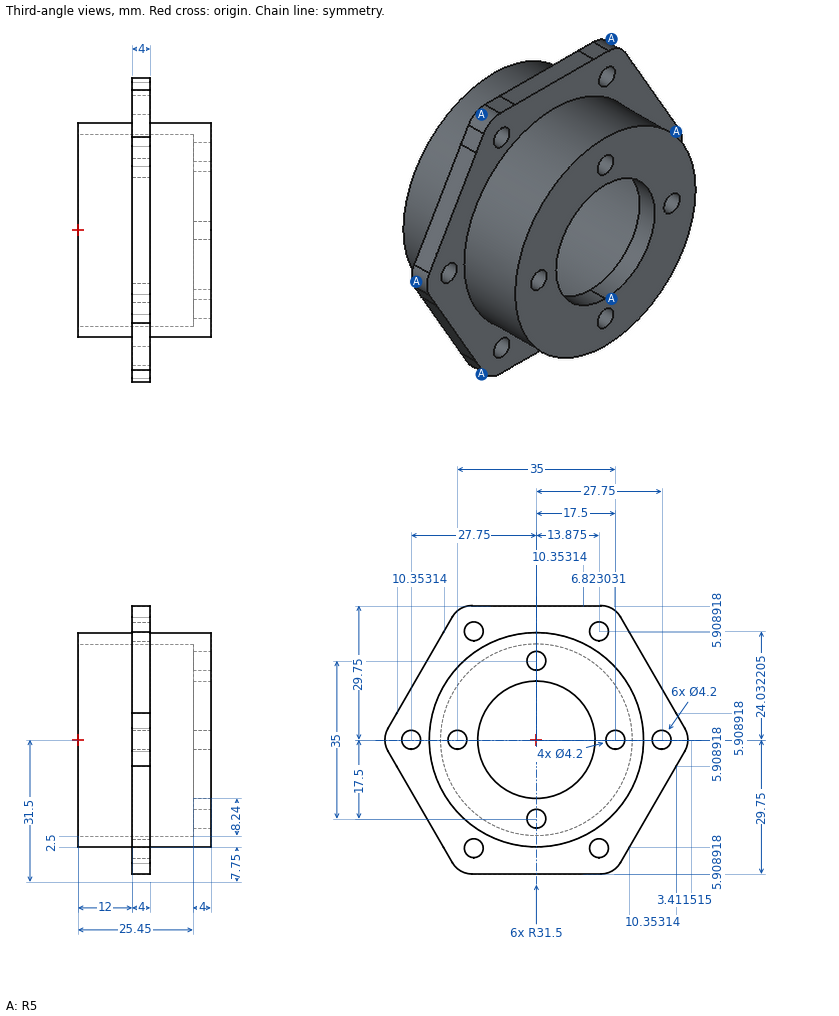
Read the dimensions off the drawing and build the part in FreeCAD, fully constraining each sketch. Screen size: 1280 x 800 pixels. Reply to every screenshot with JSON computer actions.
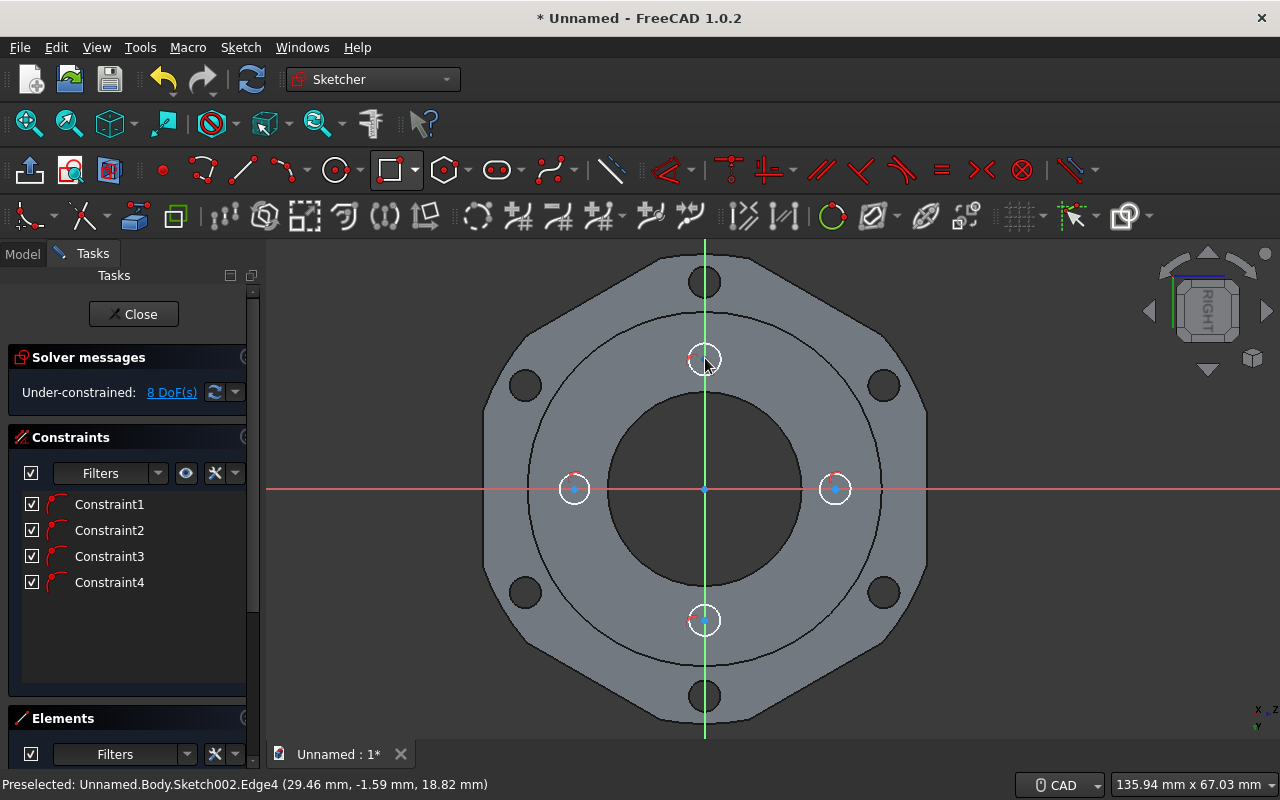
{"action": "scroll", "coordinate": [716, 609], "scroll_direction": "up", "scroll_amount": 2}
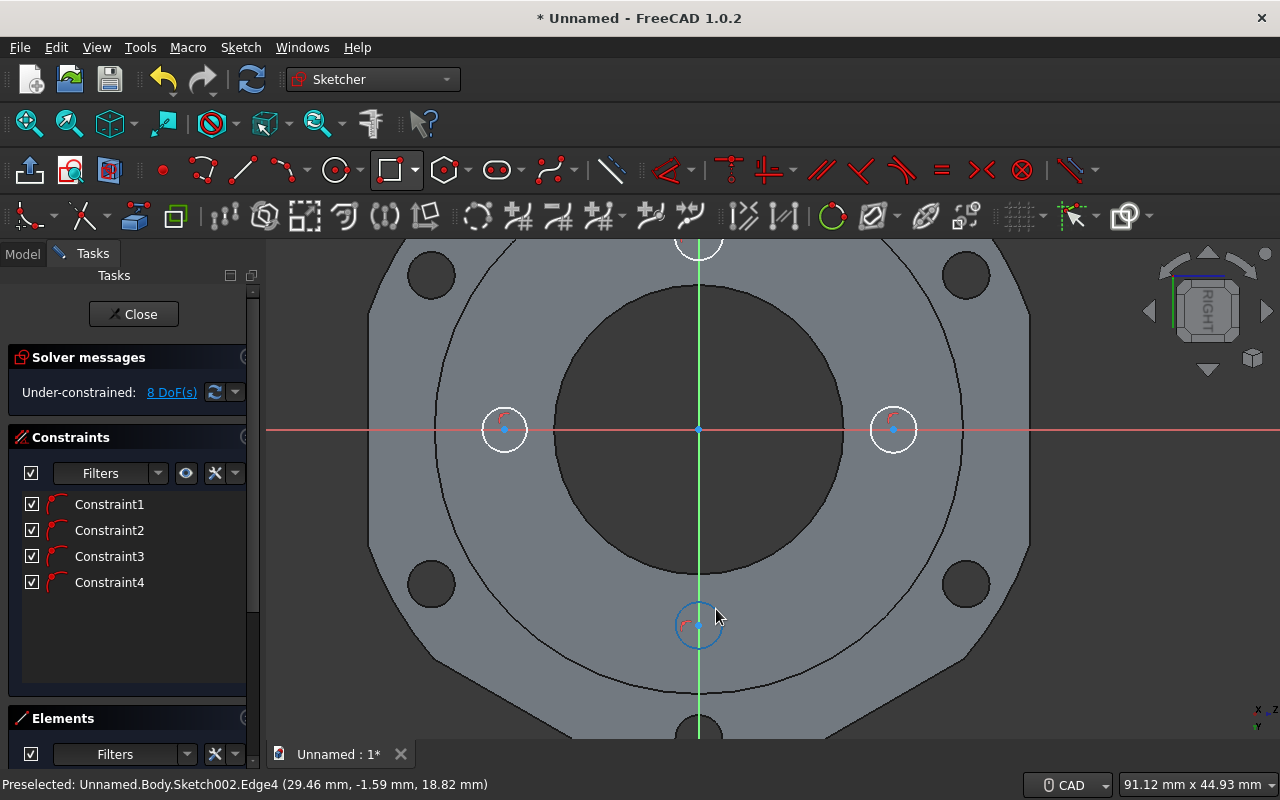
{"action": "left_click", "coordinate": [715, 609]}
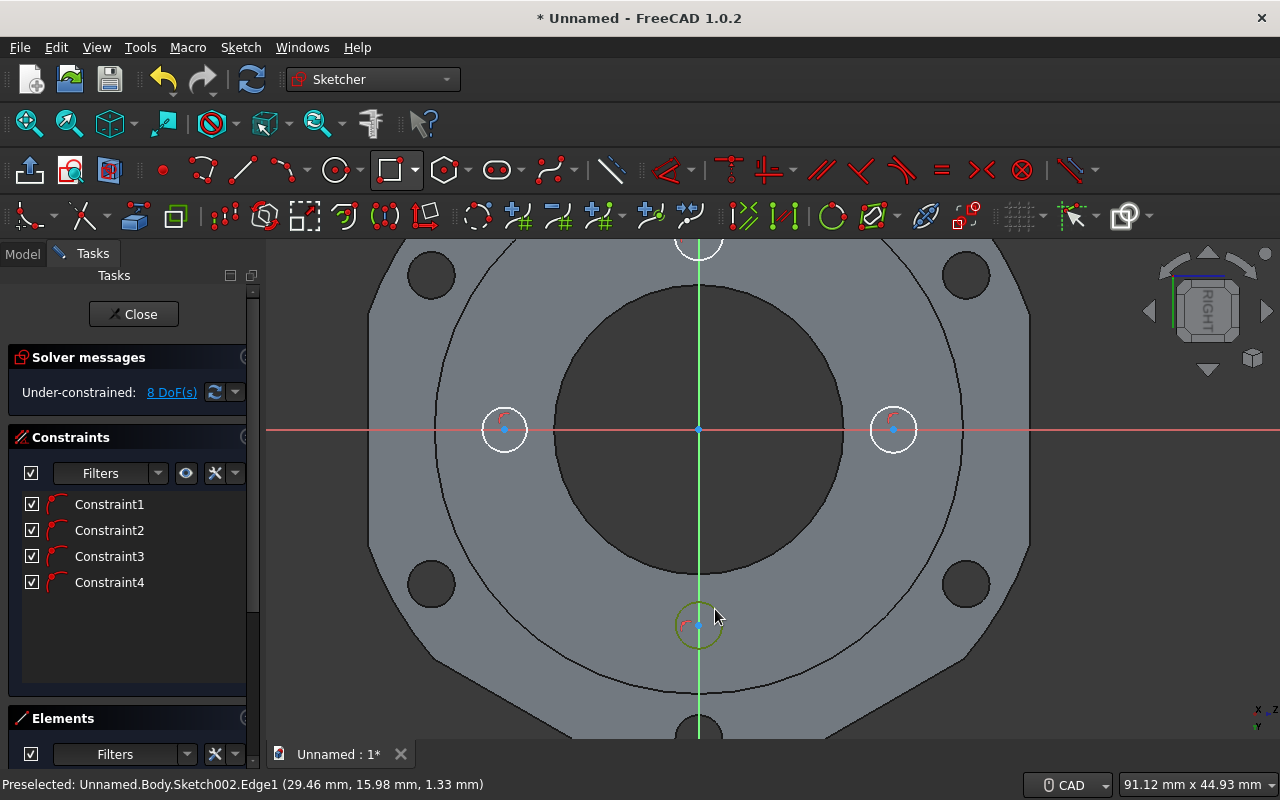
{"action": "left_click", "coordinate": [520, 414]}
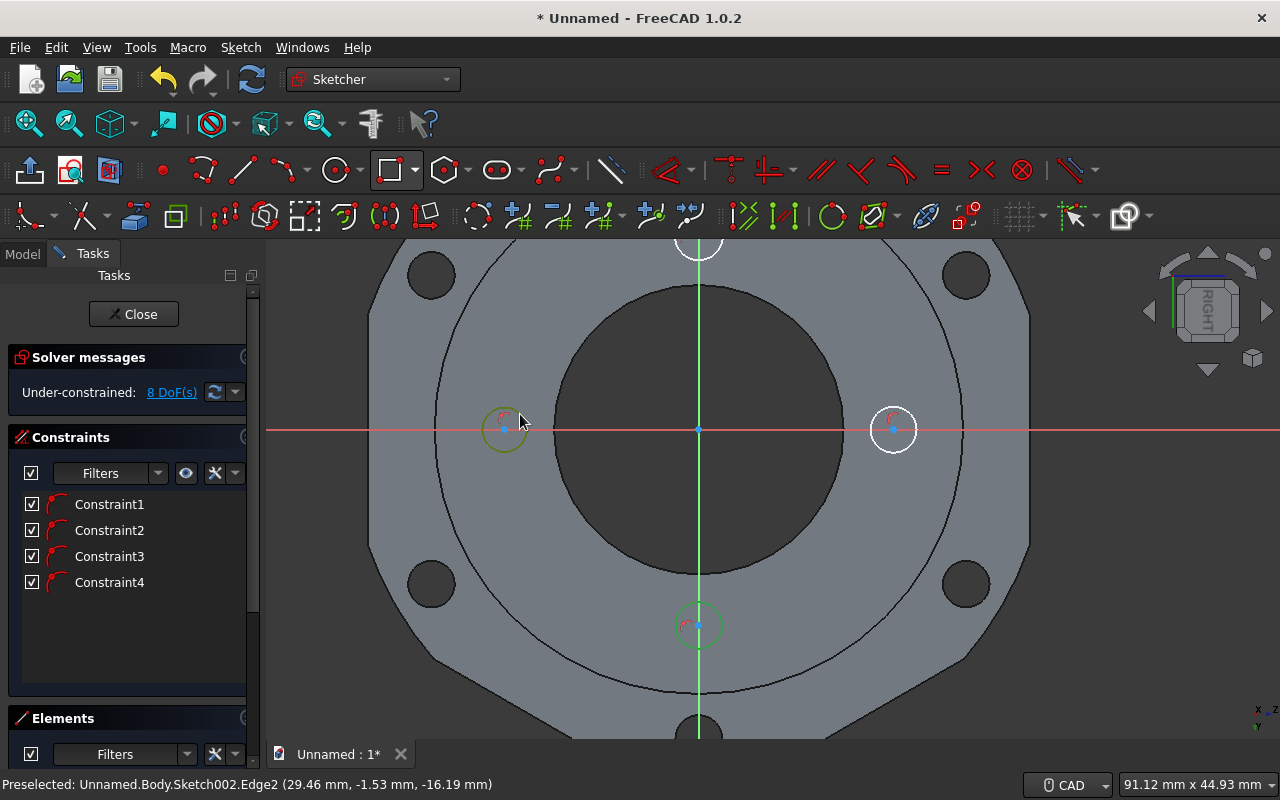
{"action": "scroll", "coordinate": [716, 609], "scroll_direction": "down", "scroll_amount": 2}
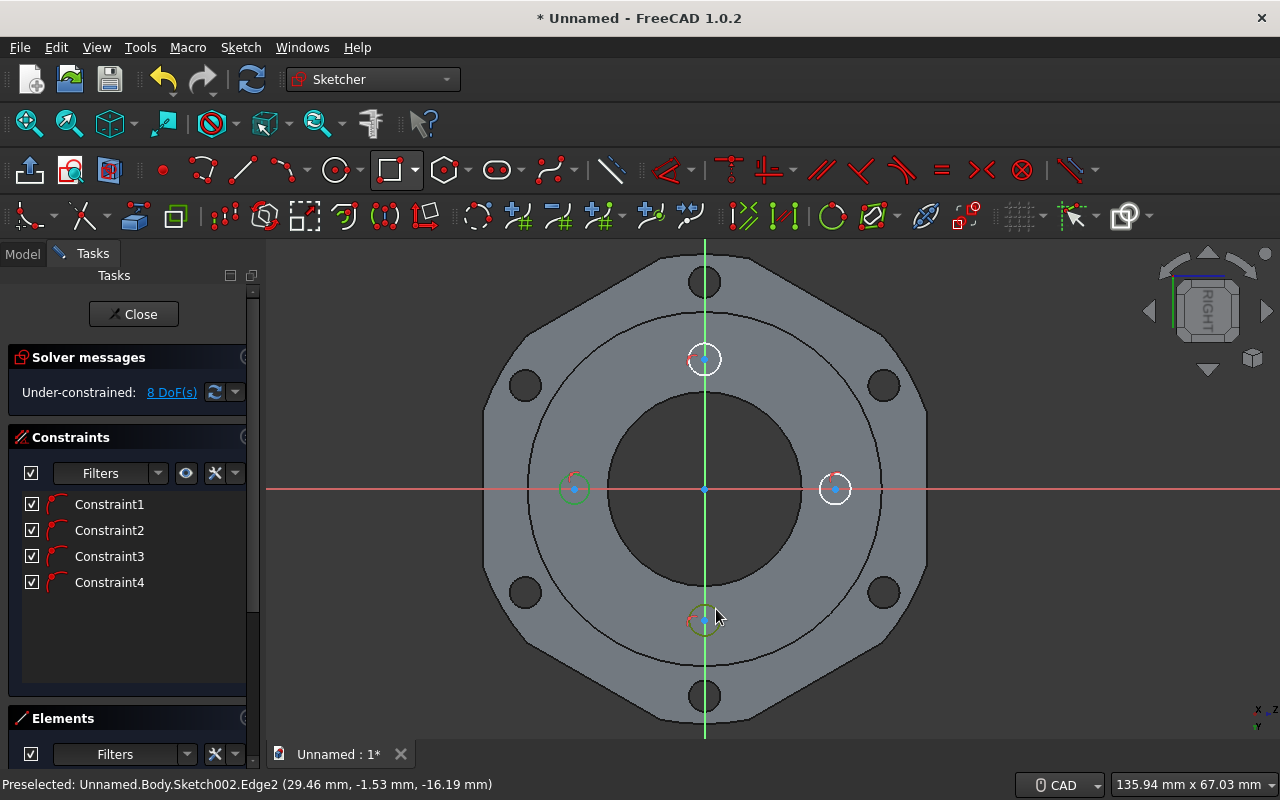
{"action": "scroll", "coordinate": [716, 348], "scroll_direction": "up", "scroll_amount": 2}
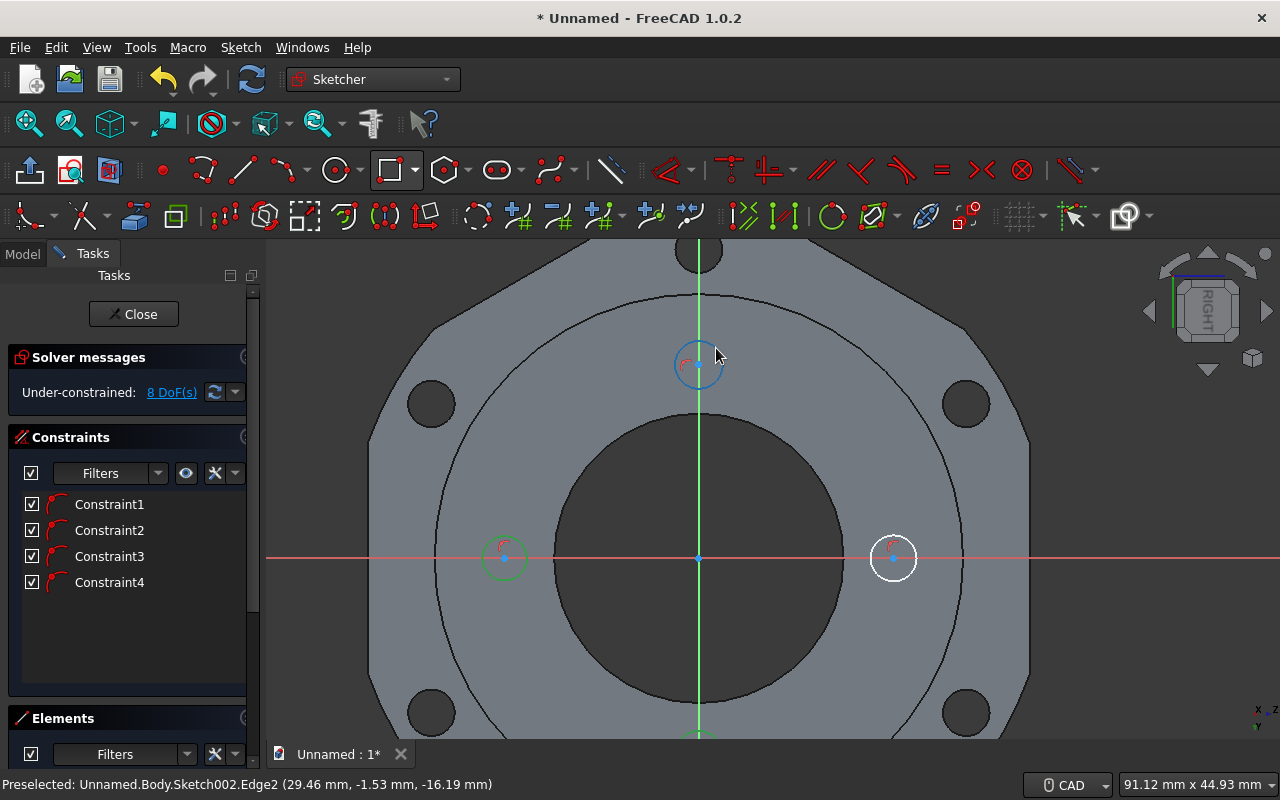
{"action": "left_click", "coordinate": [716, 348]}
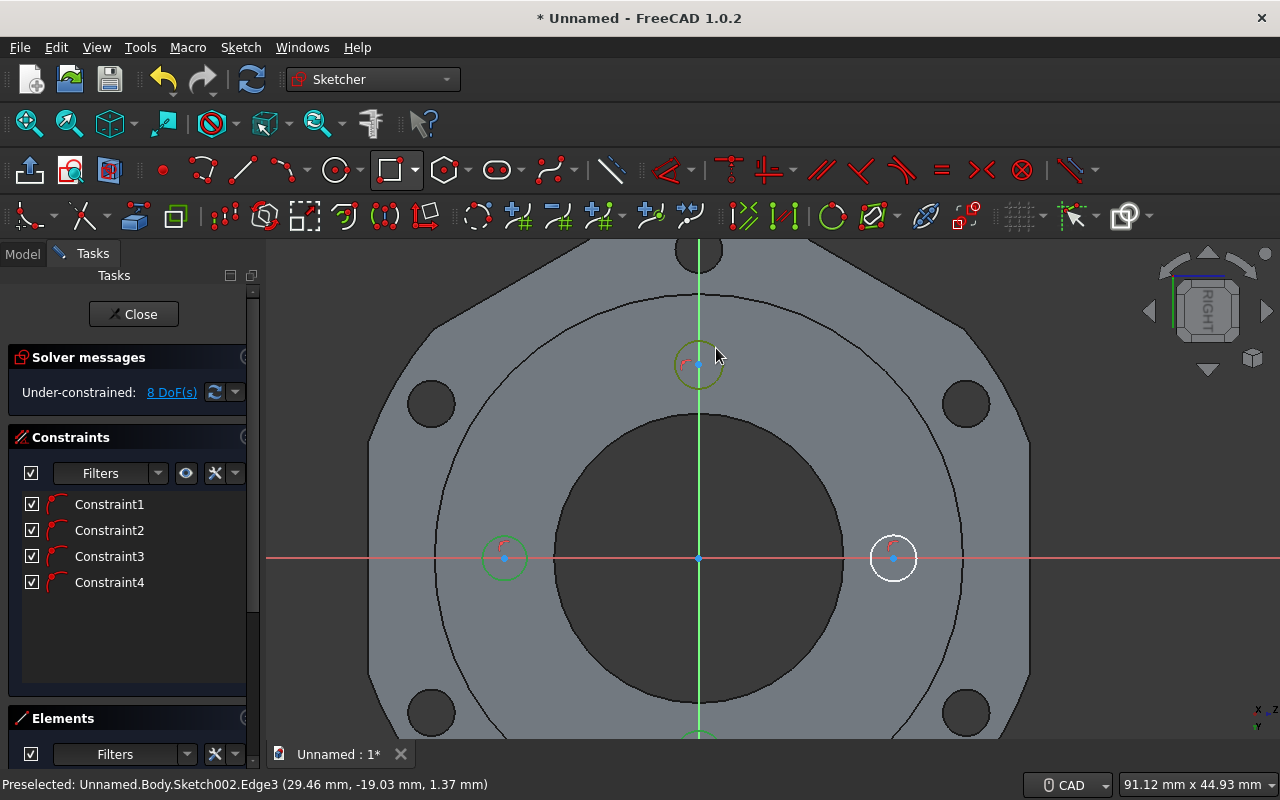
{"action": "left_click", "coordinate": [910, 542]}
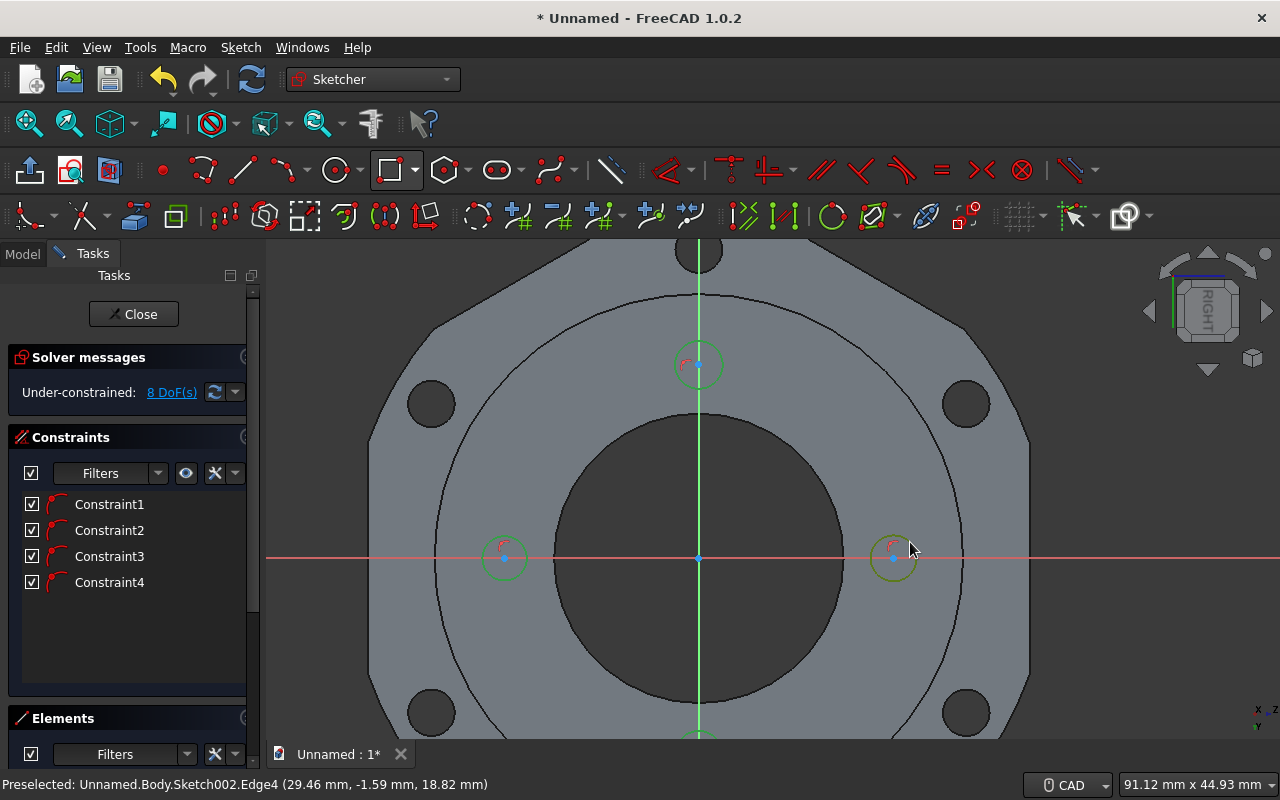
{"action": "key", "text": "e"}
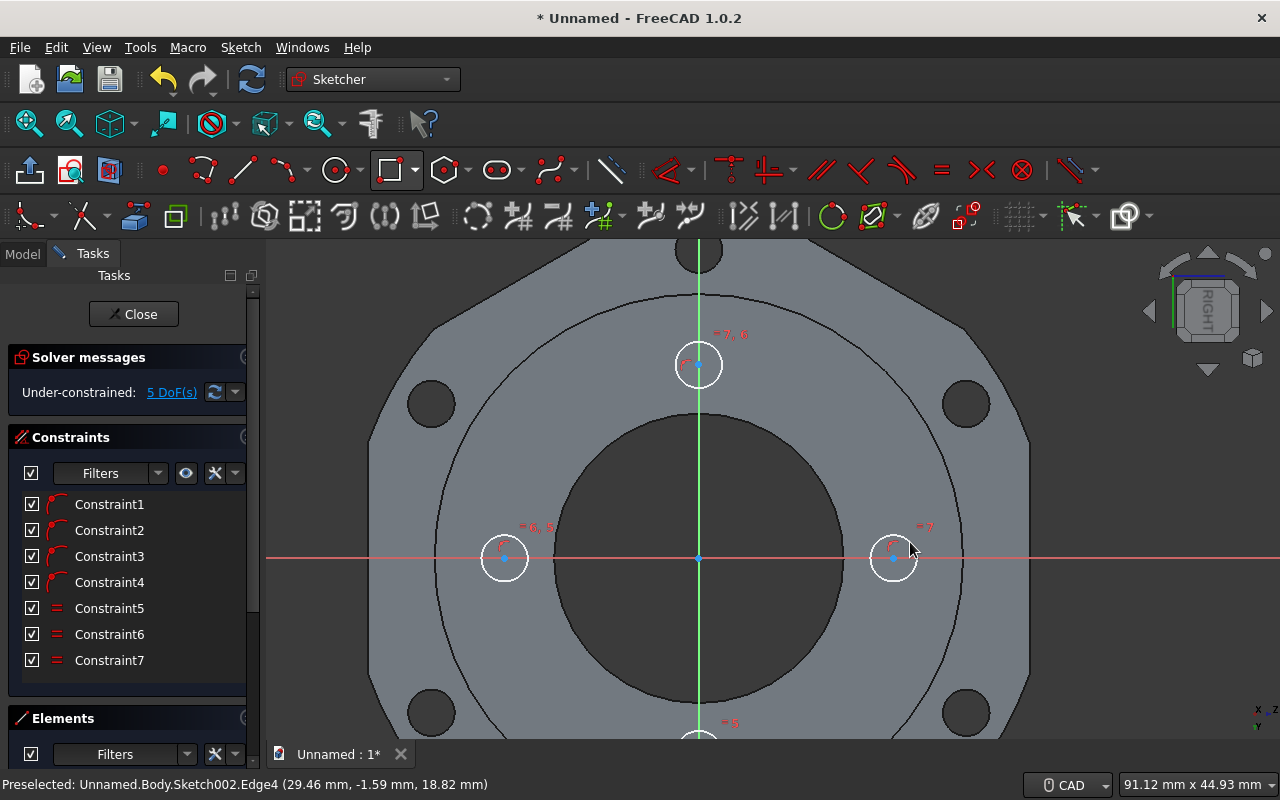
{"action": "key", "text": "d"}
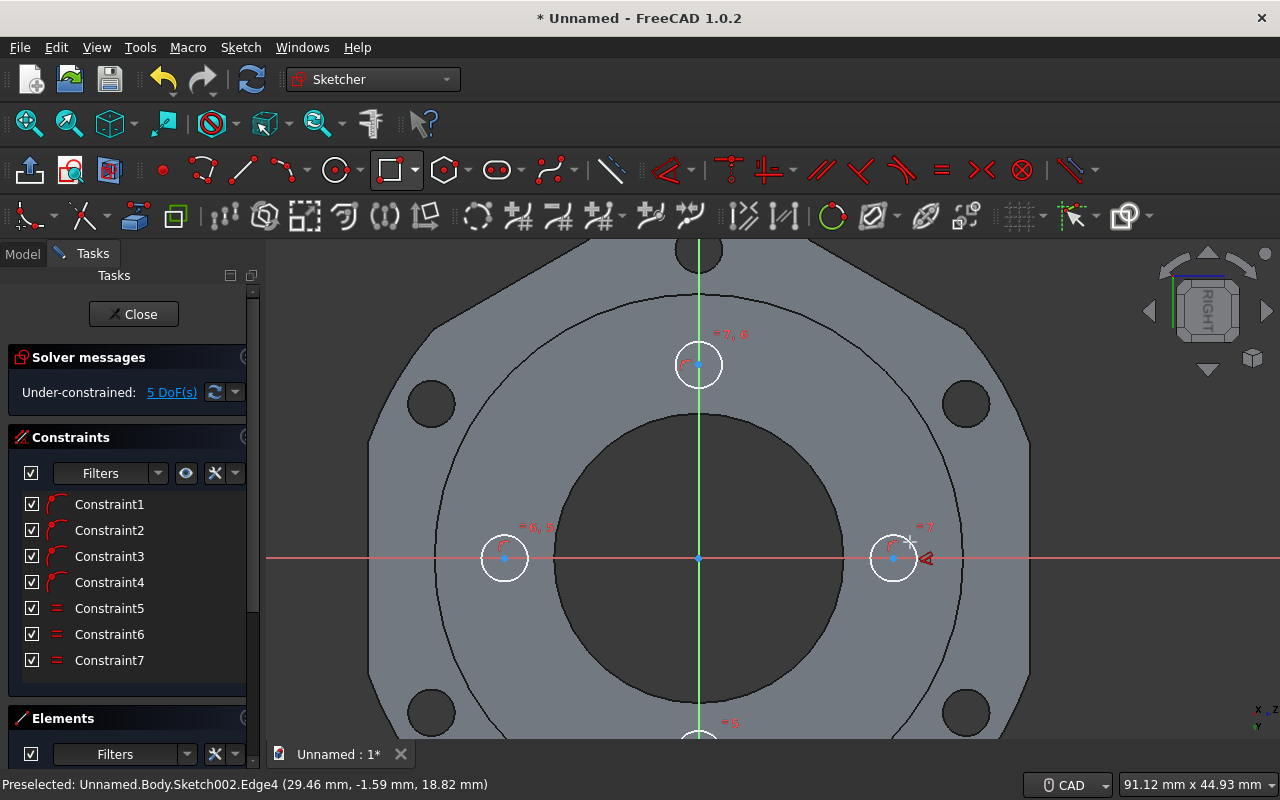
{"action": "scroll", "coordinate": [716, 348], "scroll_direction": "down", "scroll_amount": 2}